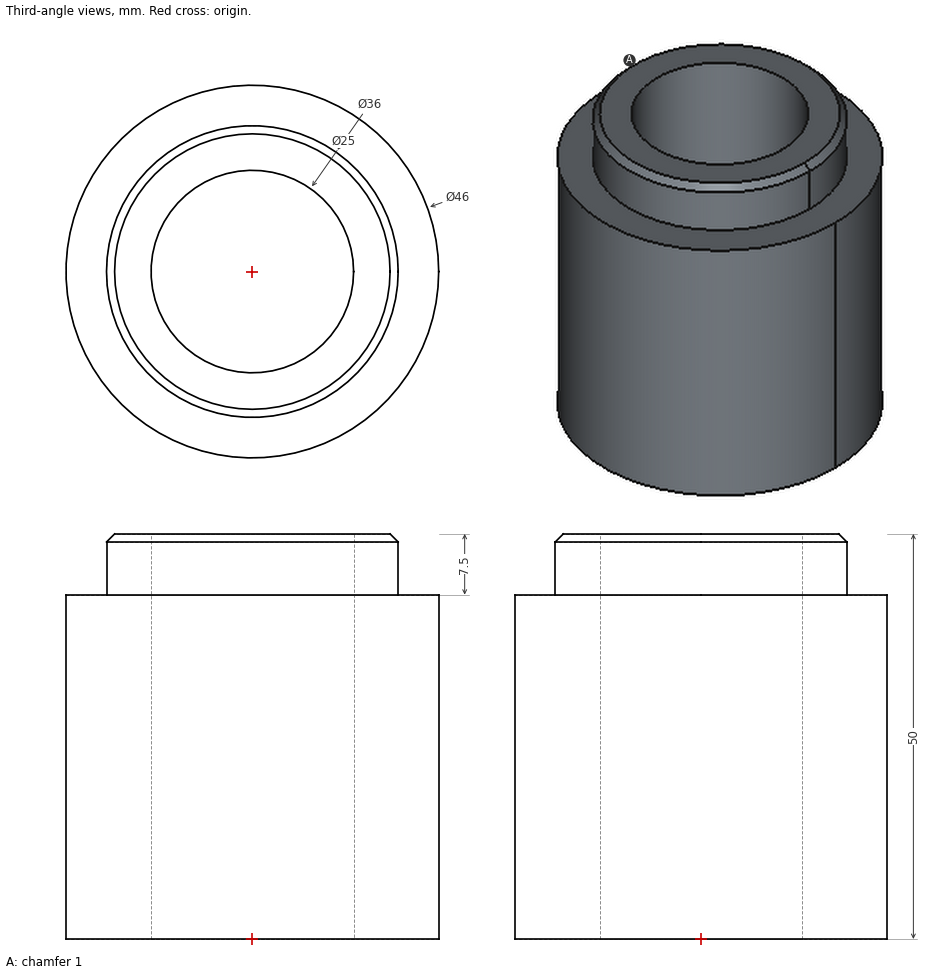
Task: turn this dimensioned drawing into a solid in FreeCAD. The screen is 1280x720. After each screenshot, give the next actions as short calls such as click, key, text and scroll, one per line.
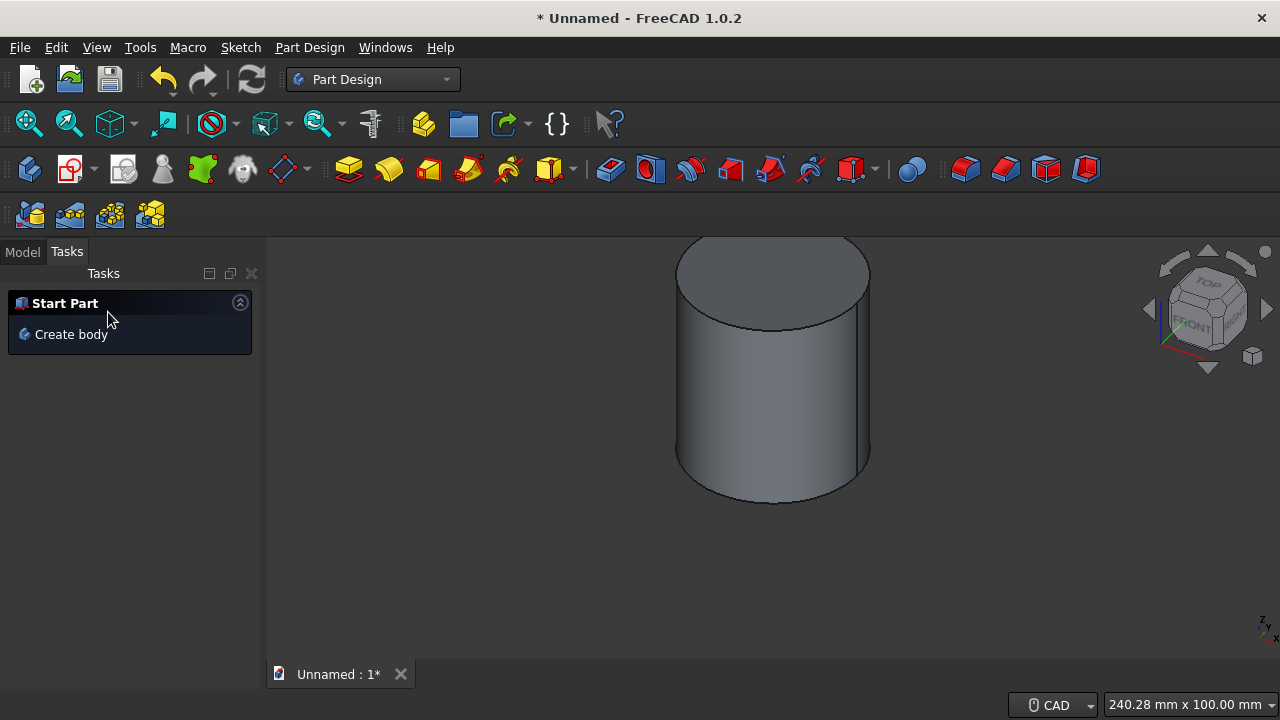
key(v)
key(f)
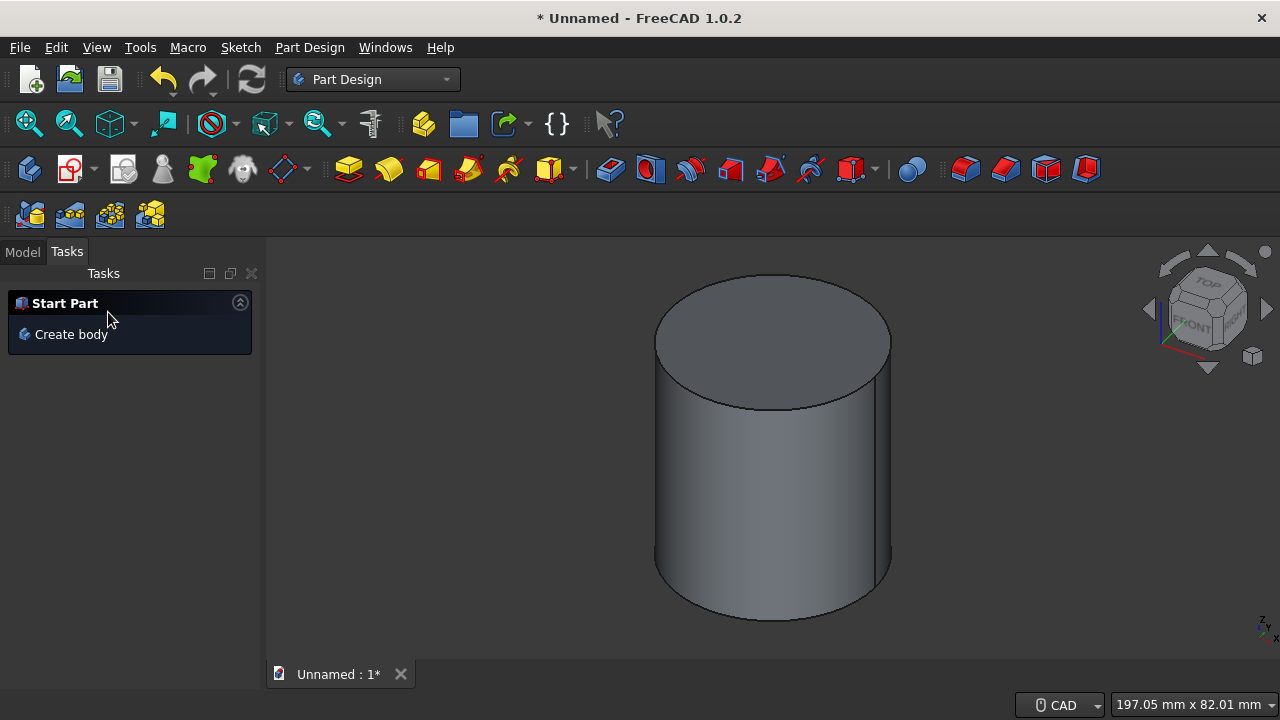
click(23, 251)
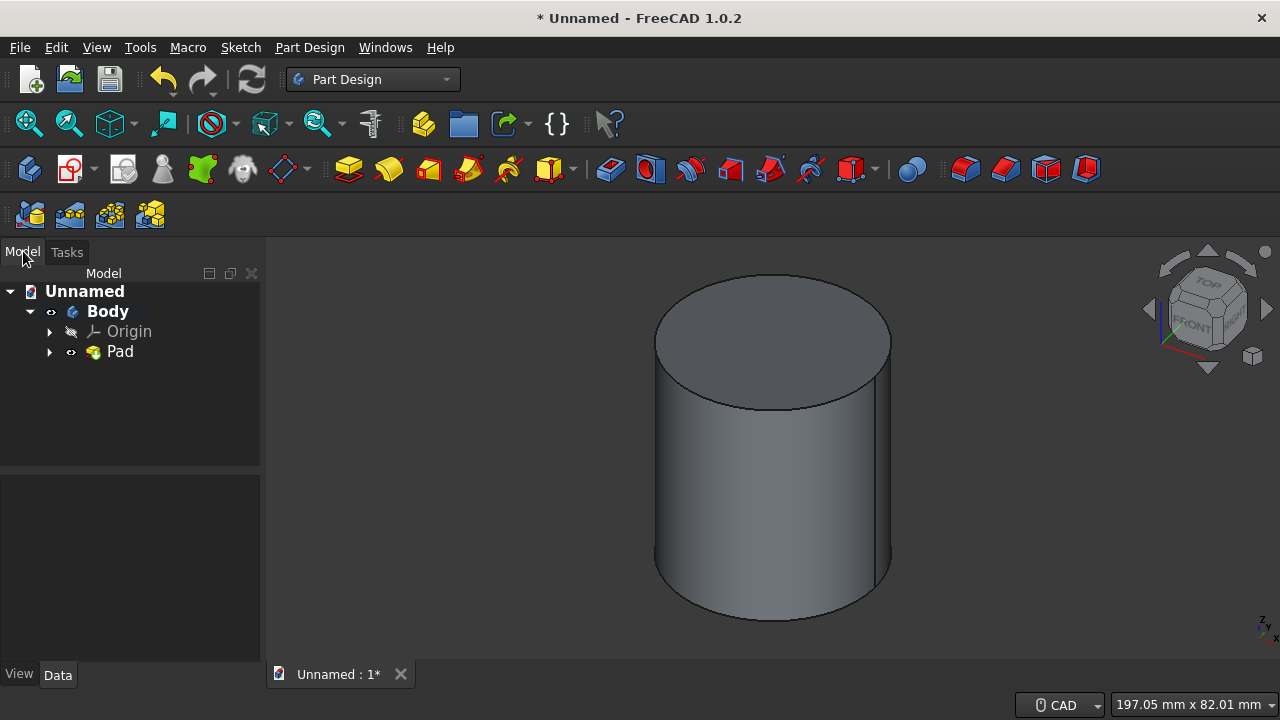
click(50, 332)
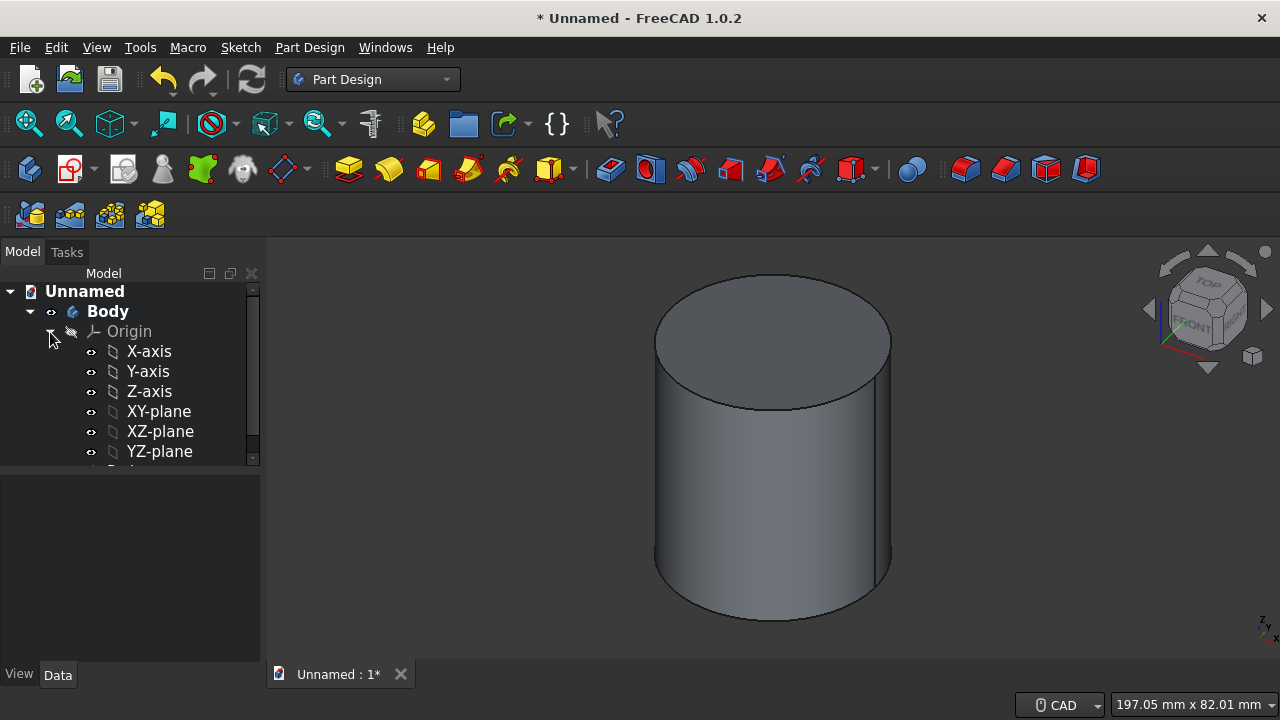
click(136, 412)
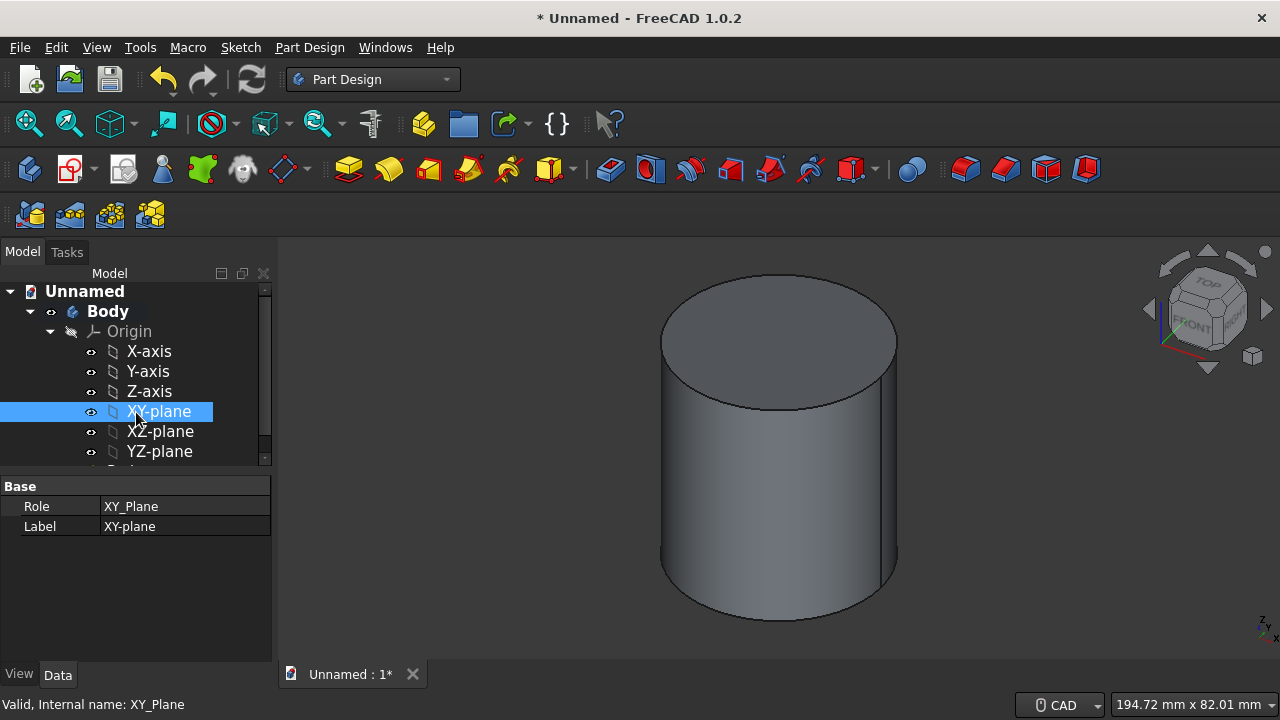
click(284, 170)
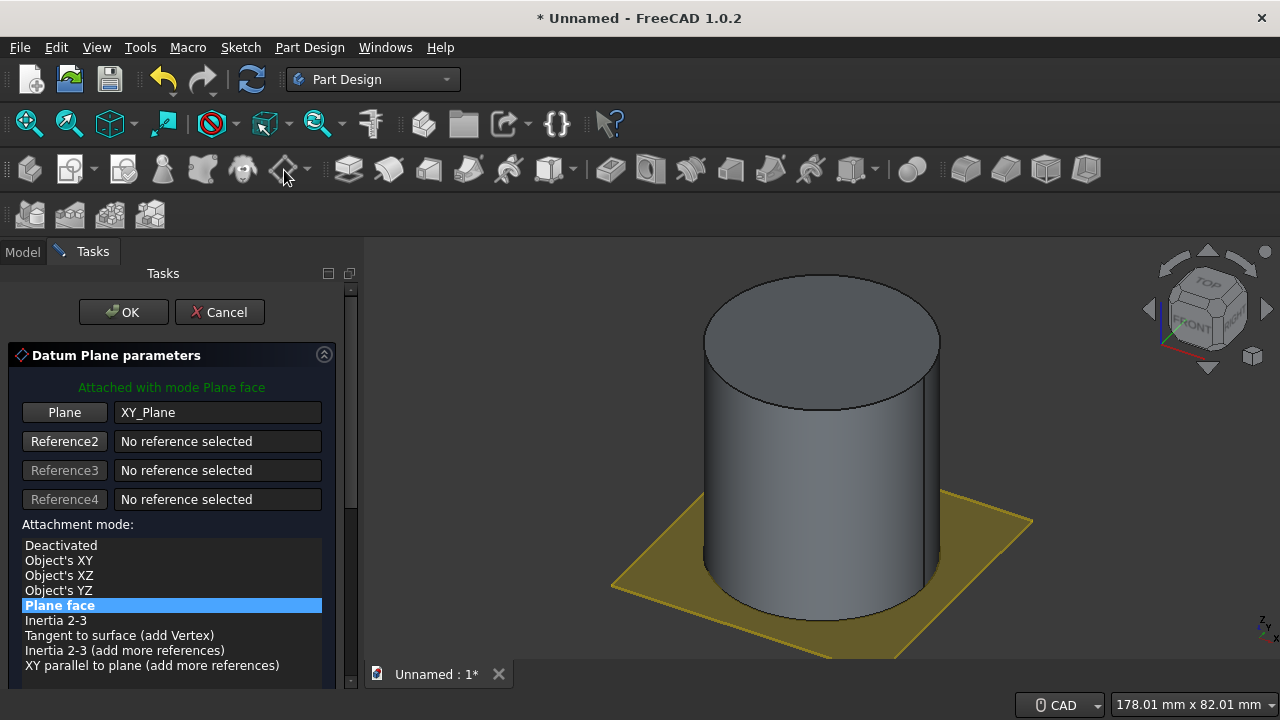
scroll(351, 486, down, 4)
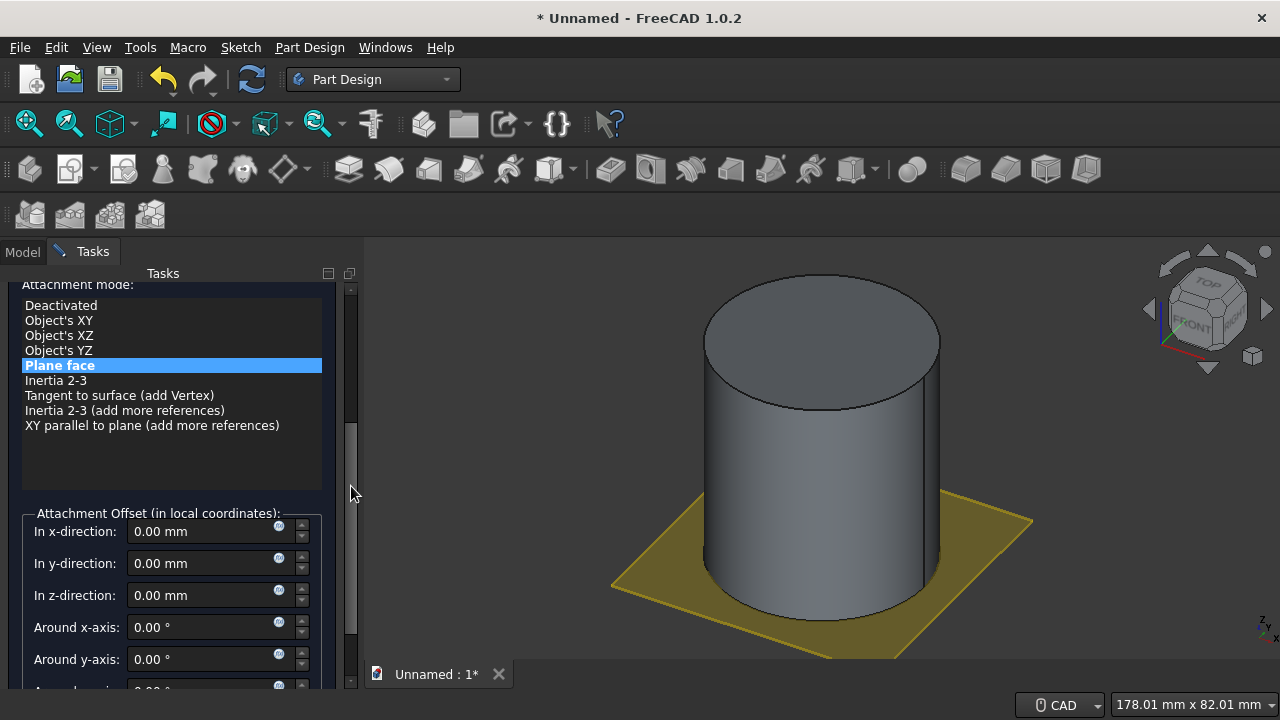
triple_click(210, 595)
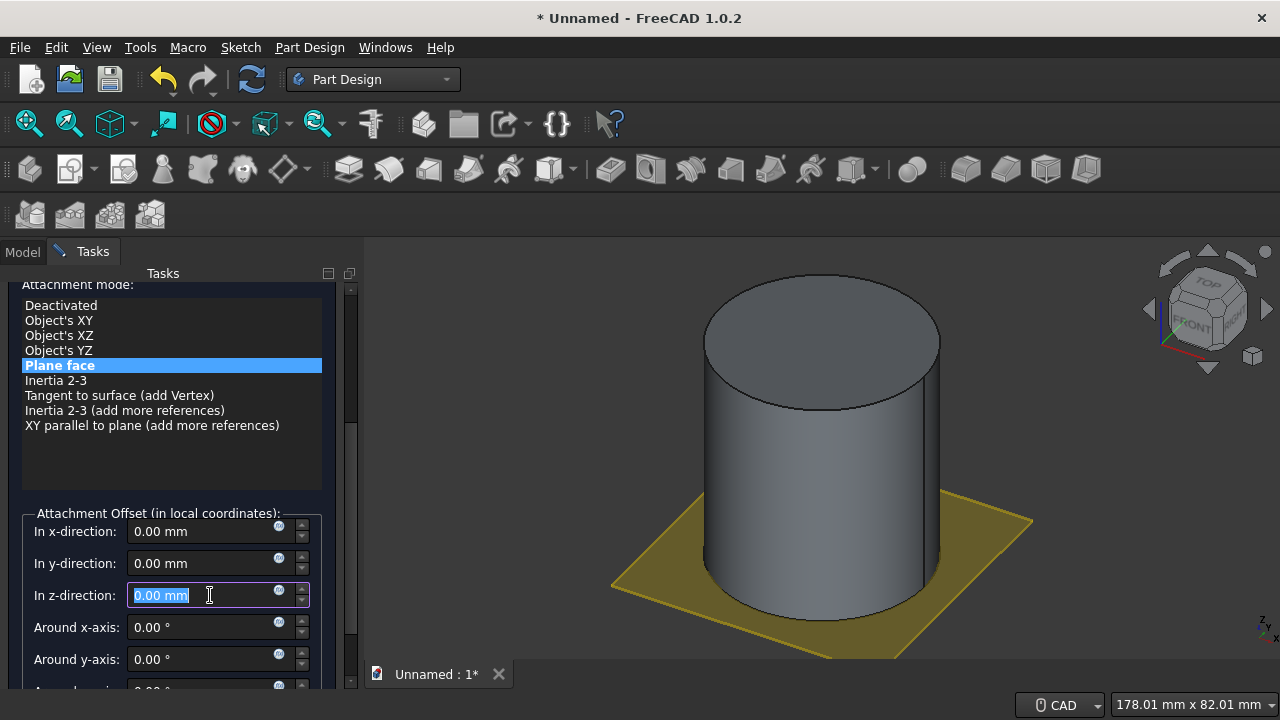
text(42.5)
key(Tab)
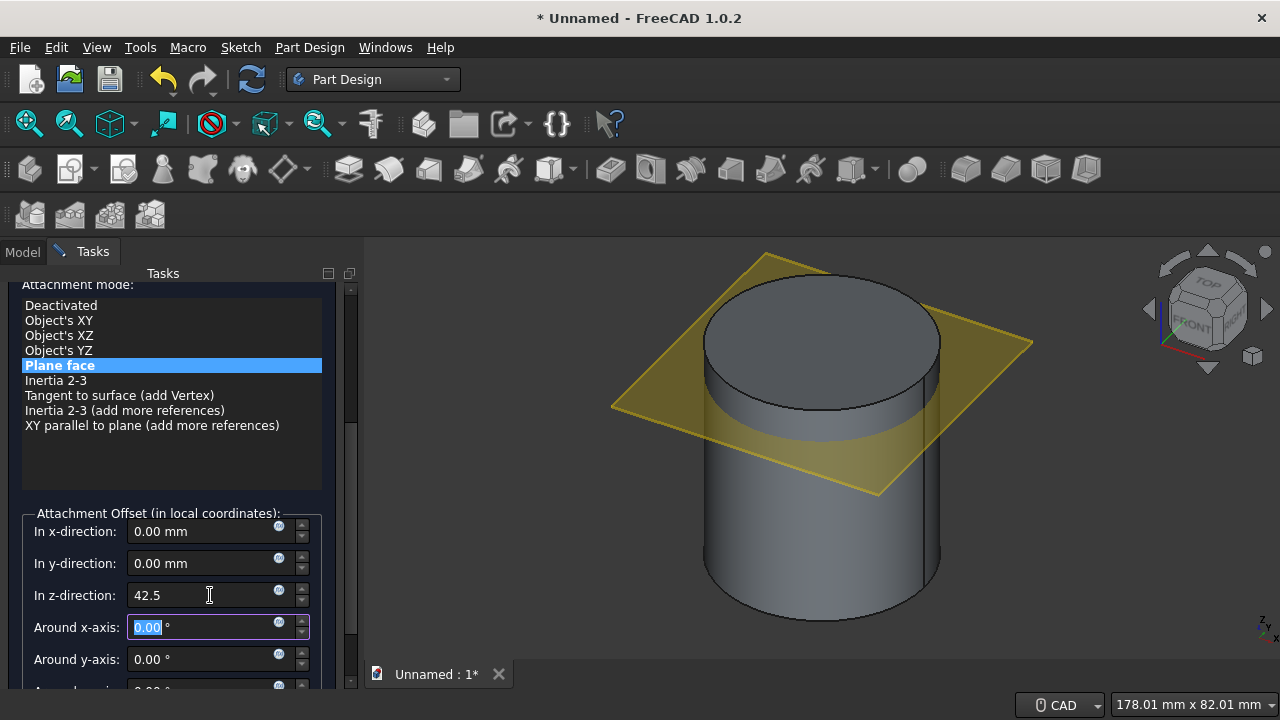
scroll(351, 486, up, 5)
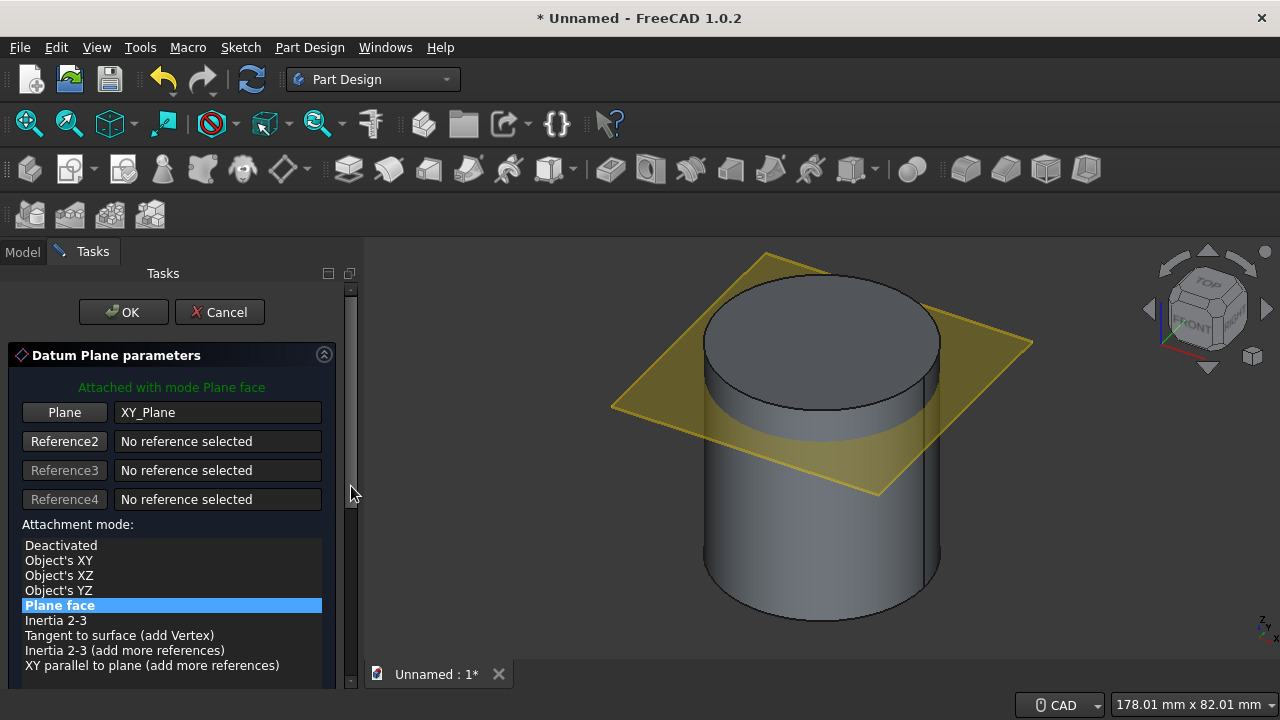
click(124, 312)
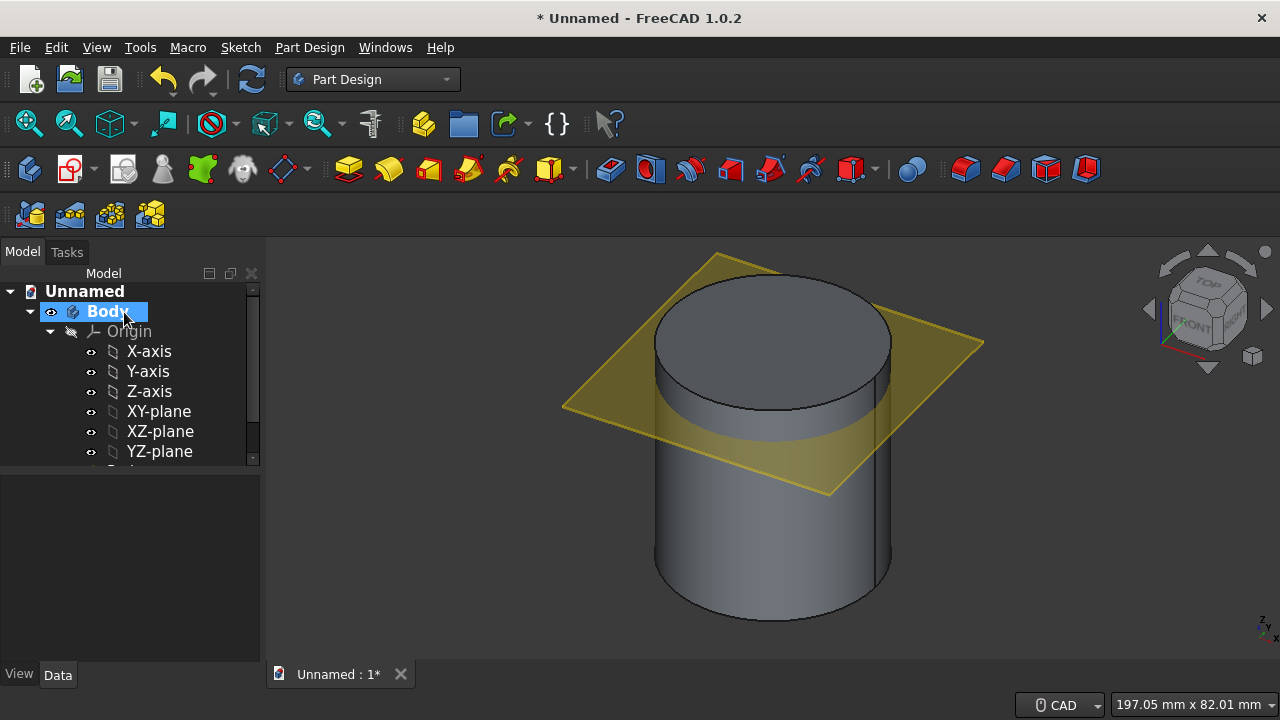
scroll(100, 367, down, 3)